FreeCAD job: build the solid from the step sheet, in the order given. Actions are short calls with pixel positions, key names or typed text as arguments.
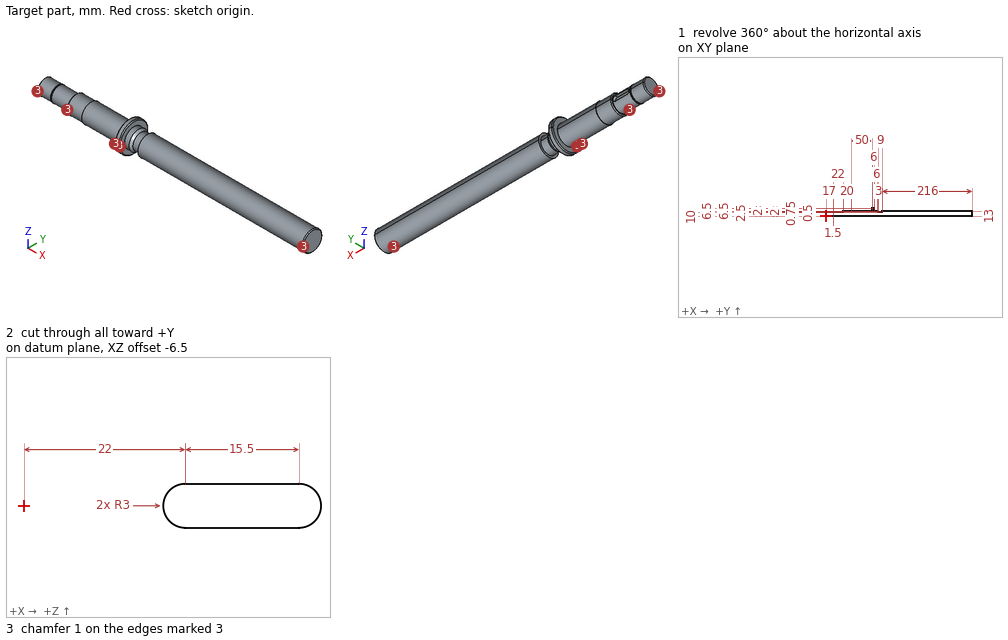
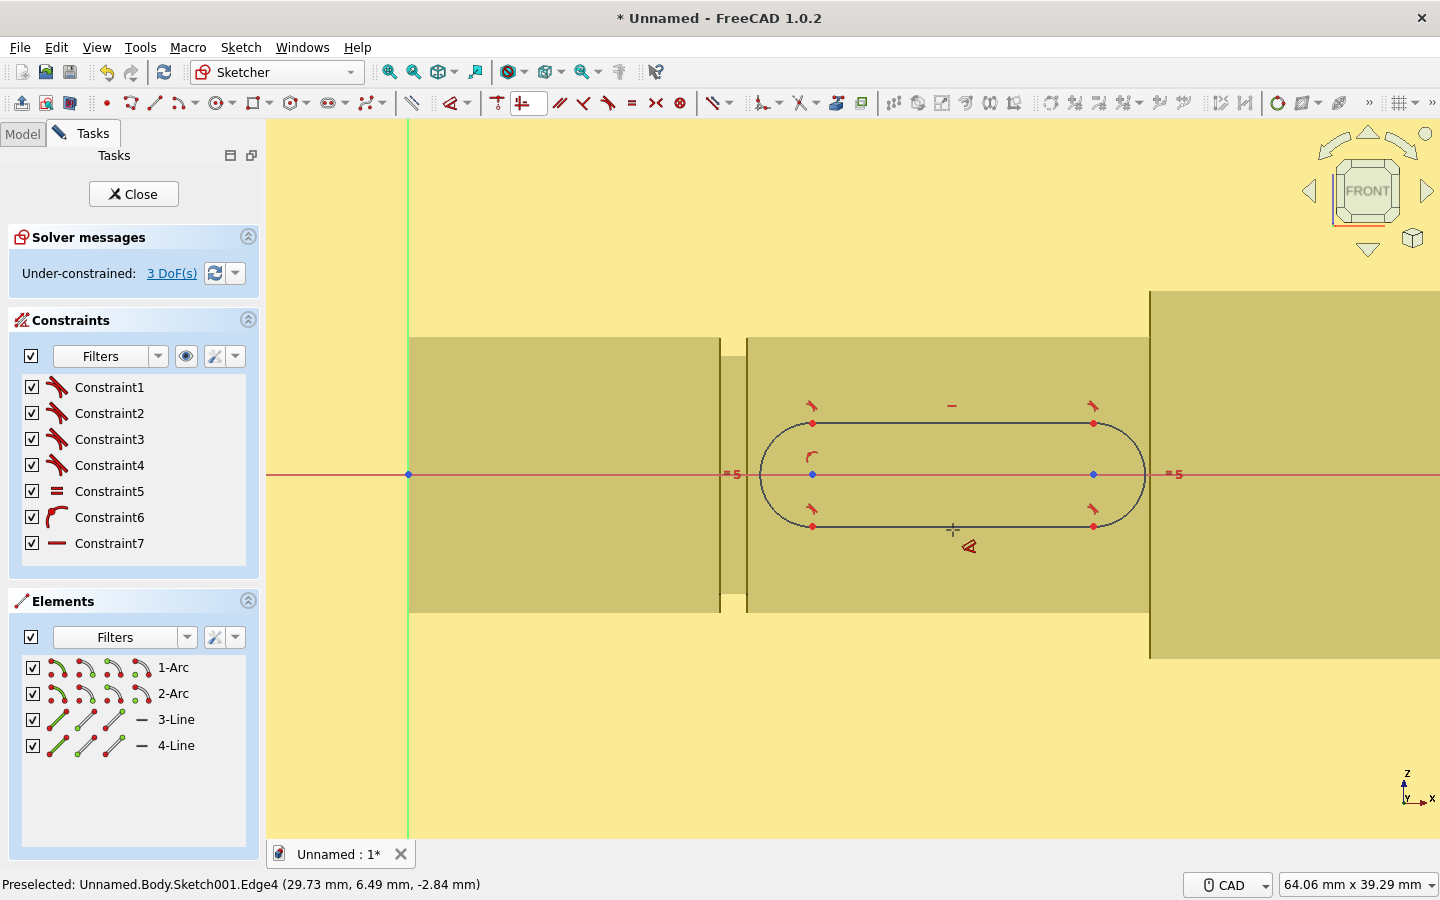
click(770, 444)
click(744, 425)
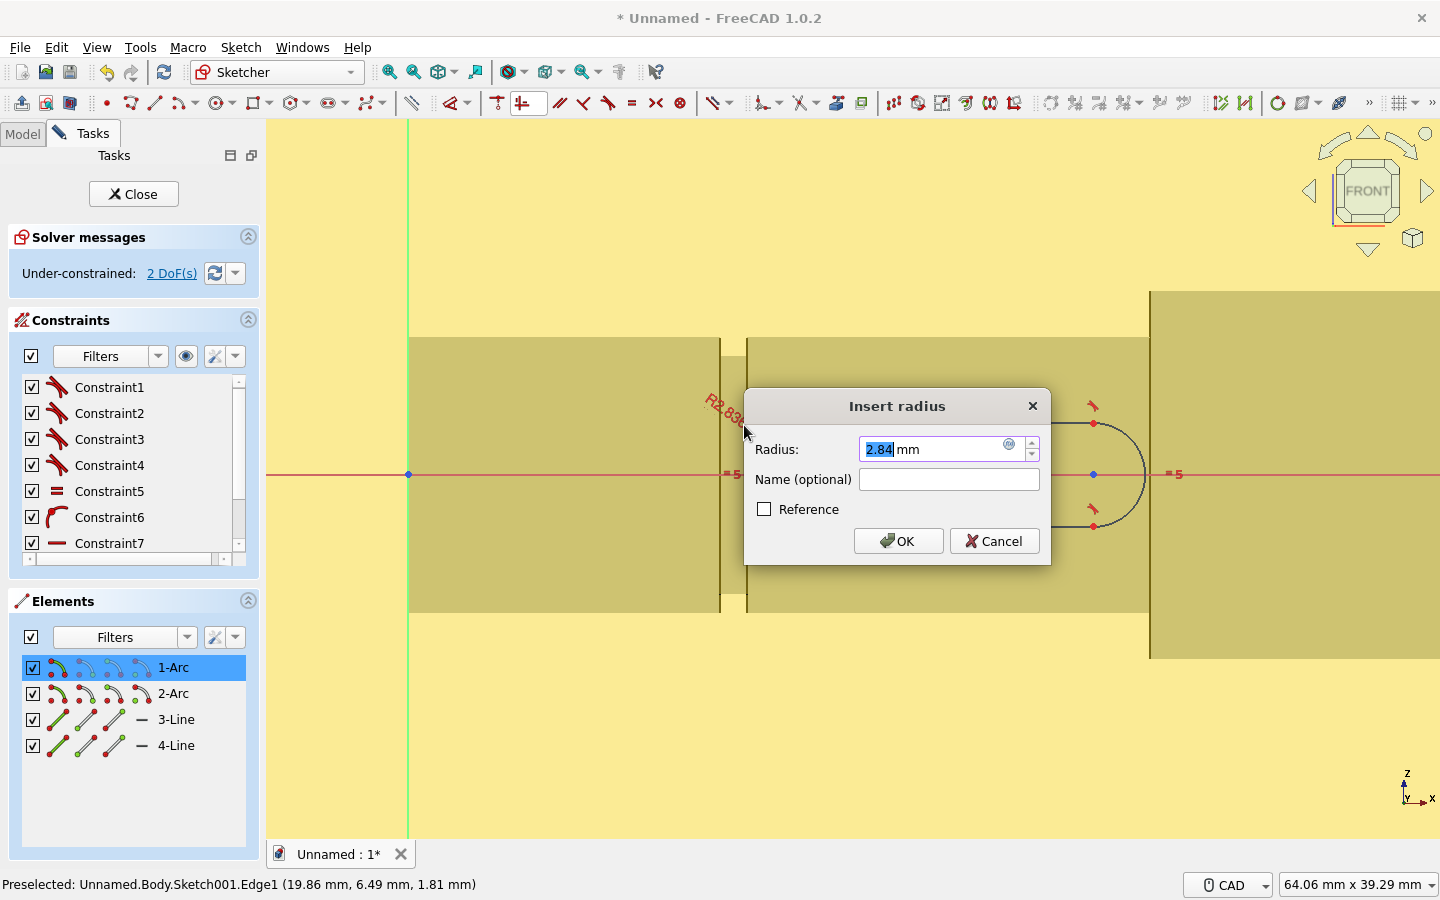
text(3)
key(Return)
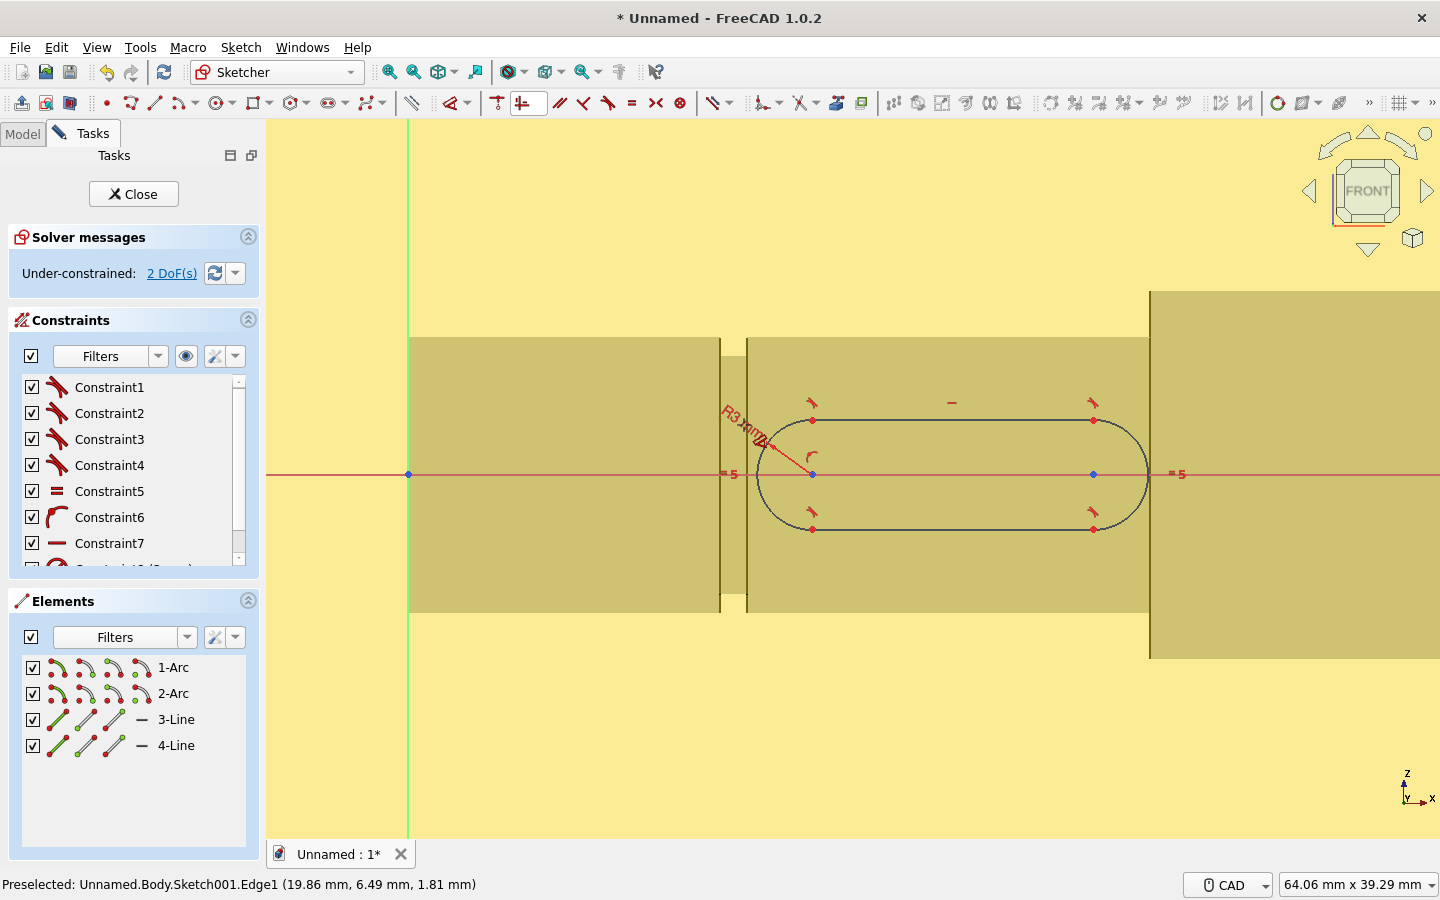
click(812, 420)
click(610, 386)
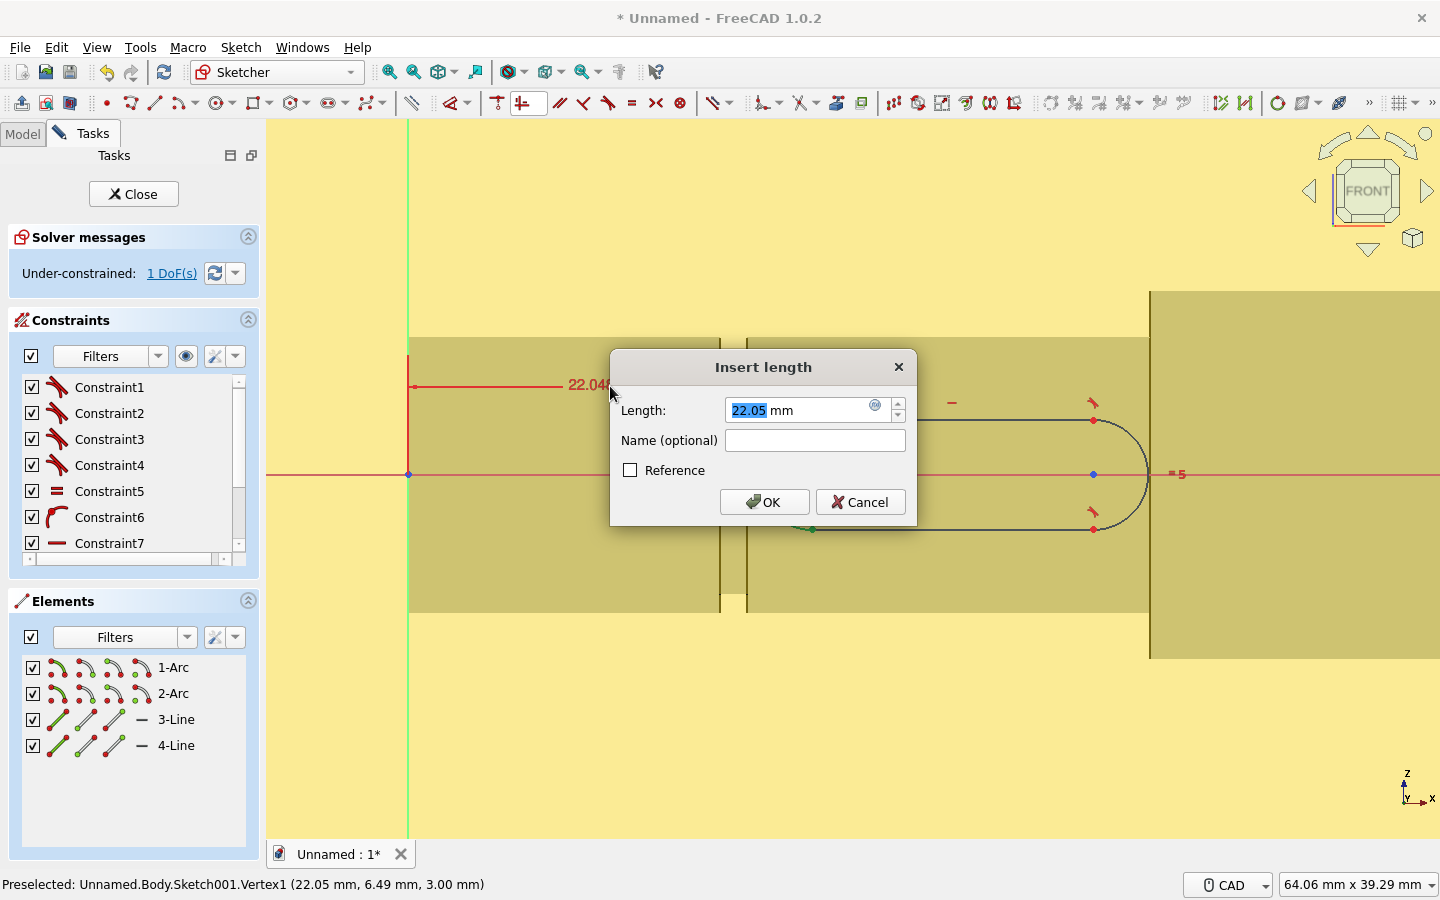
text(22)
key(Return)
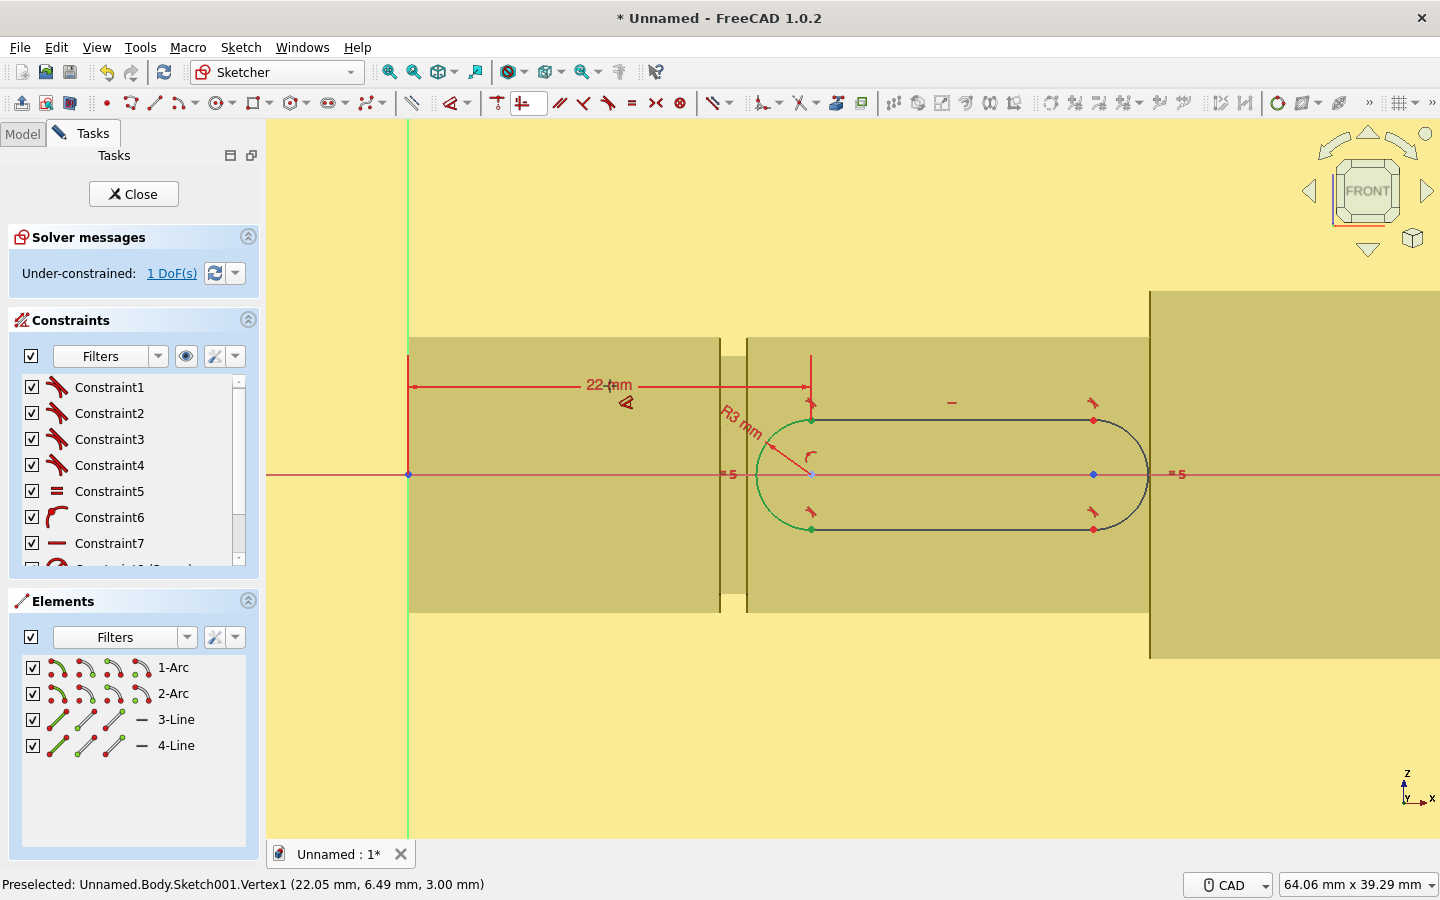
click(896, 420)
click(952, 386)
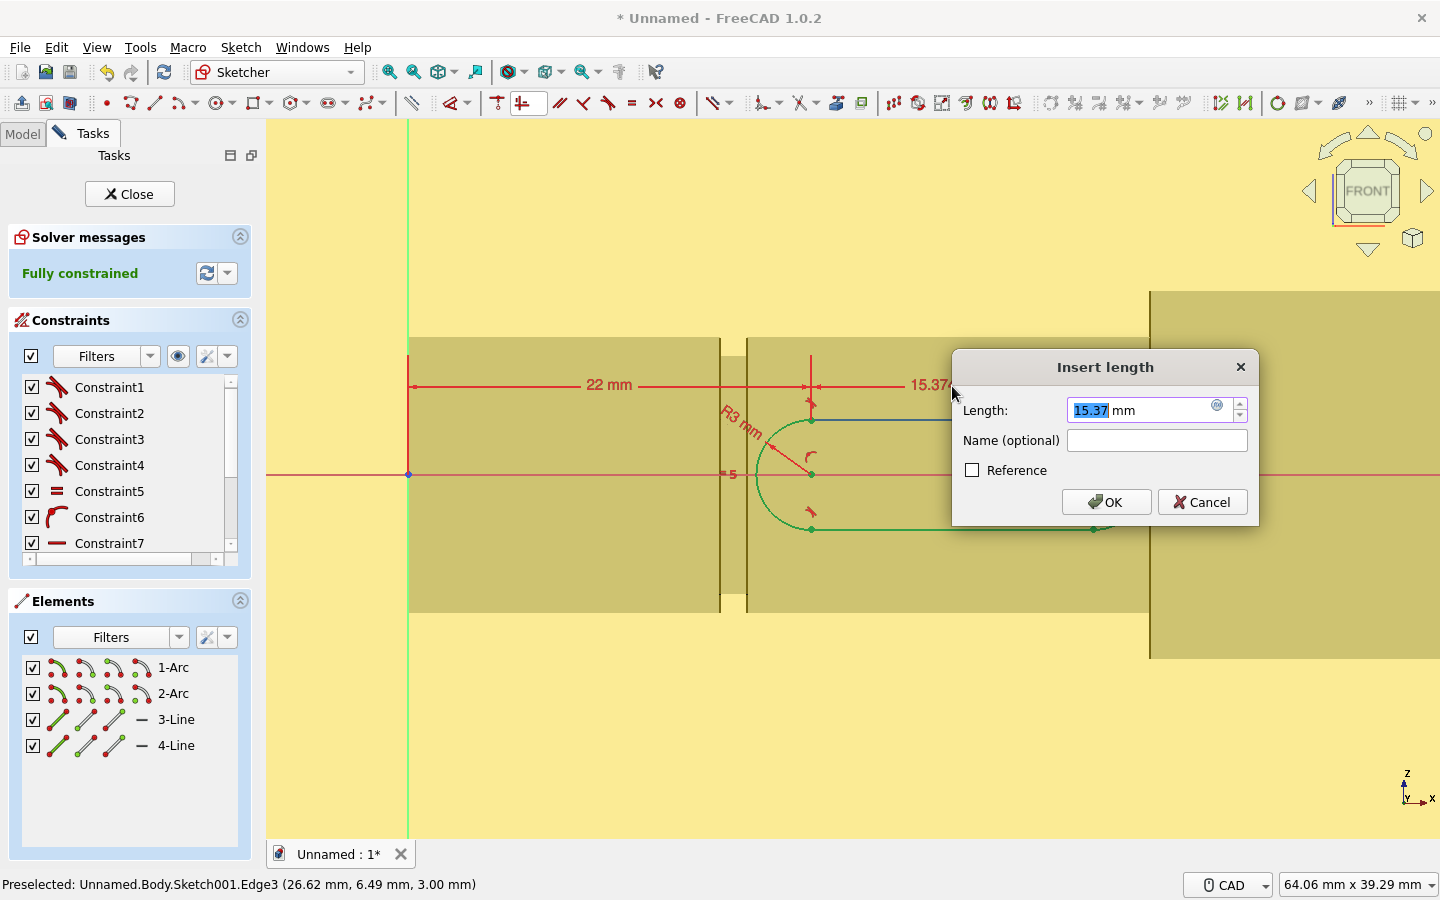
text(15.5)
key(Return)
key(Escape)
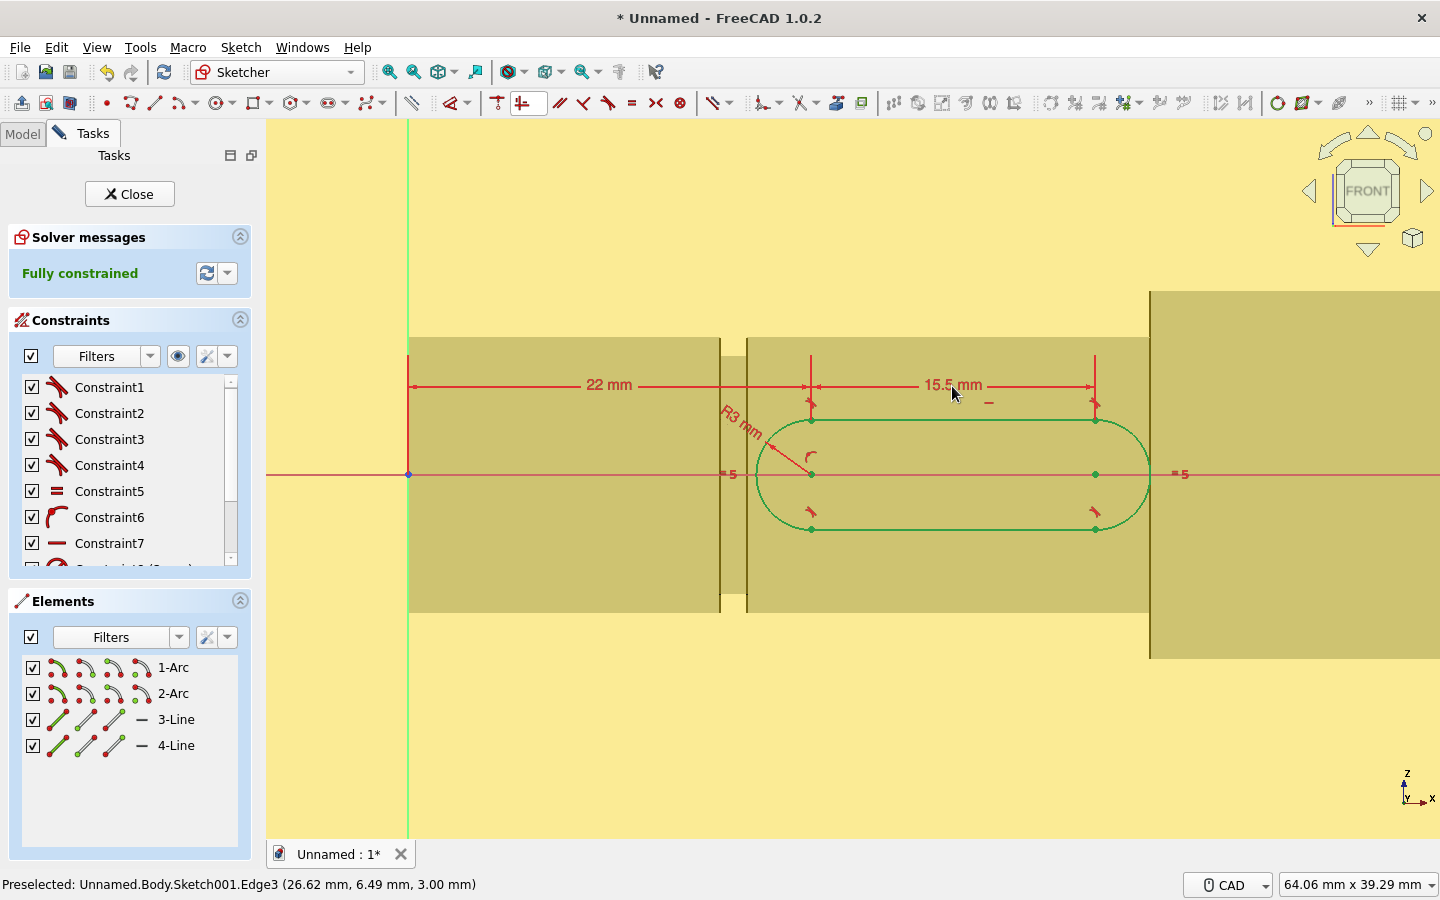
click(130, 194)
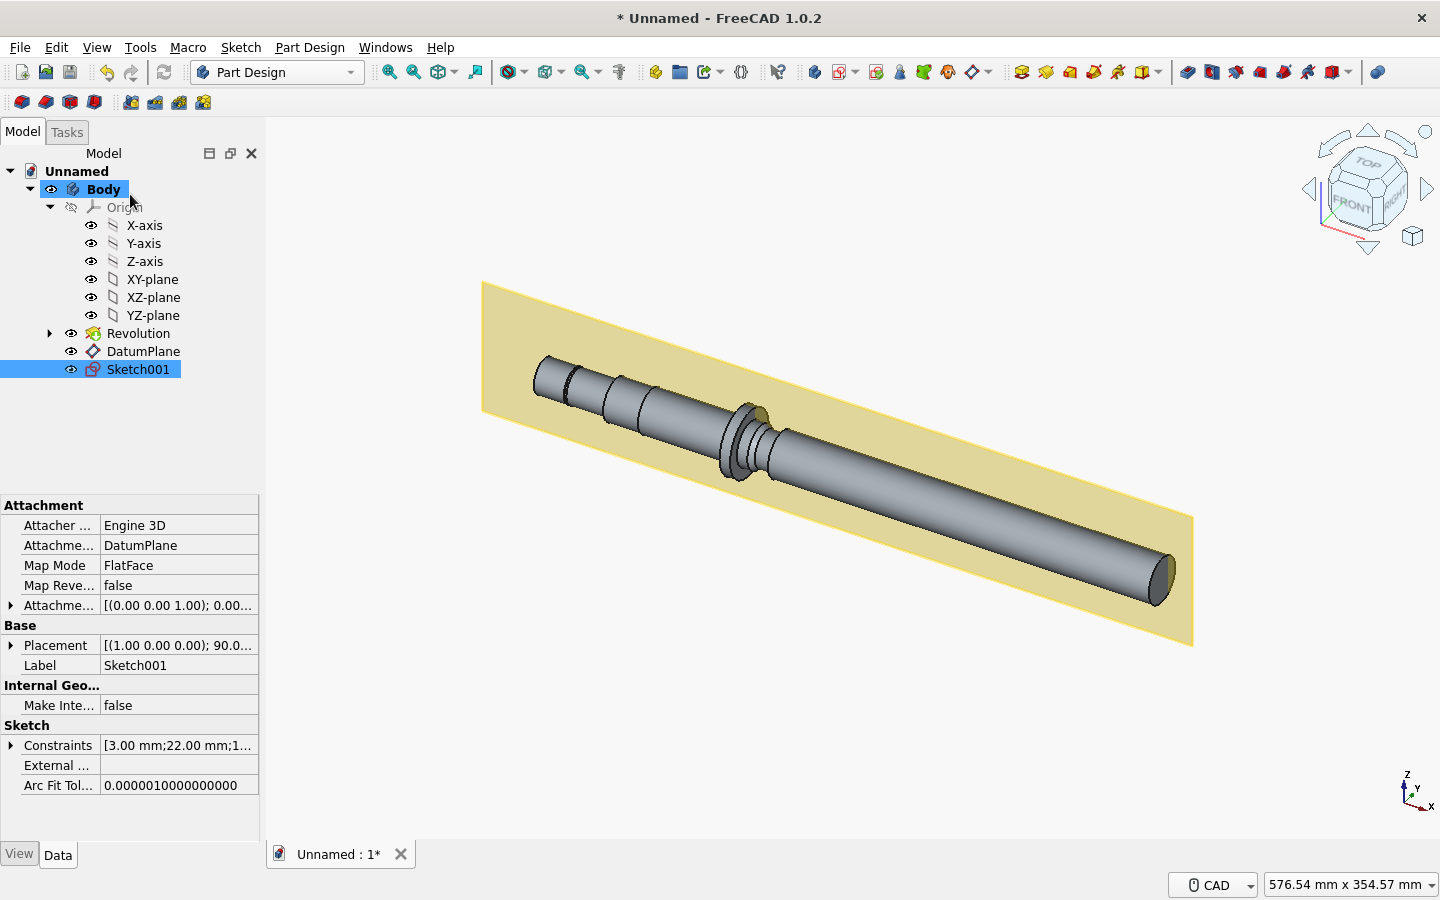
click(1188, 72)